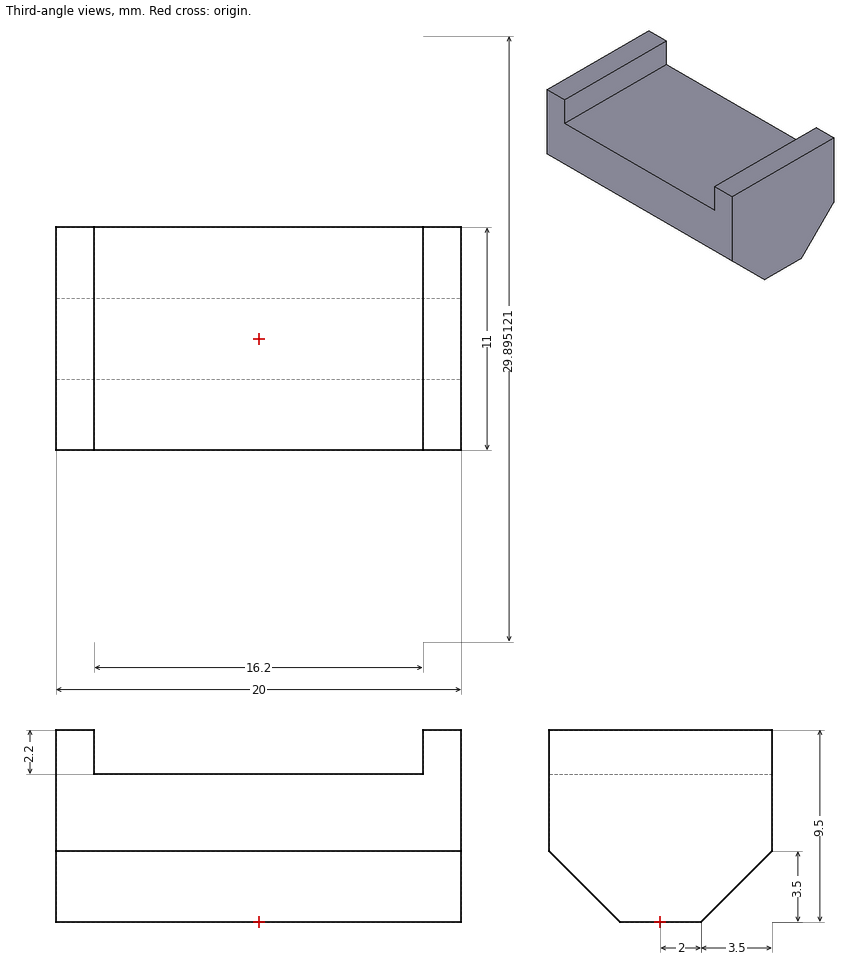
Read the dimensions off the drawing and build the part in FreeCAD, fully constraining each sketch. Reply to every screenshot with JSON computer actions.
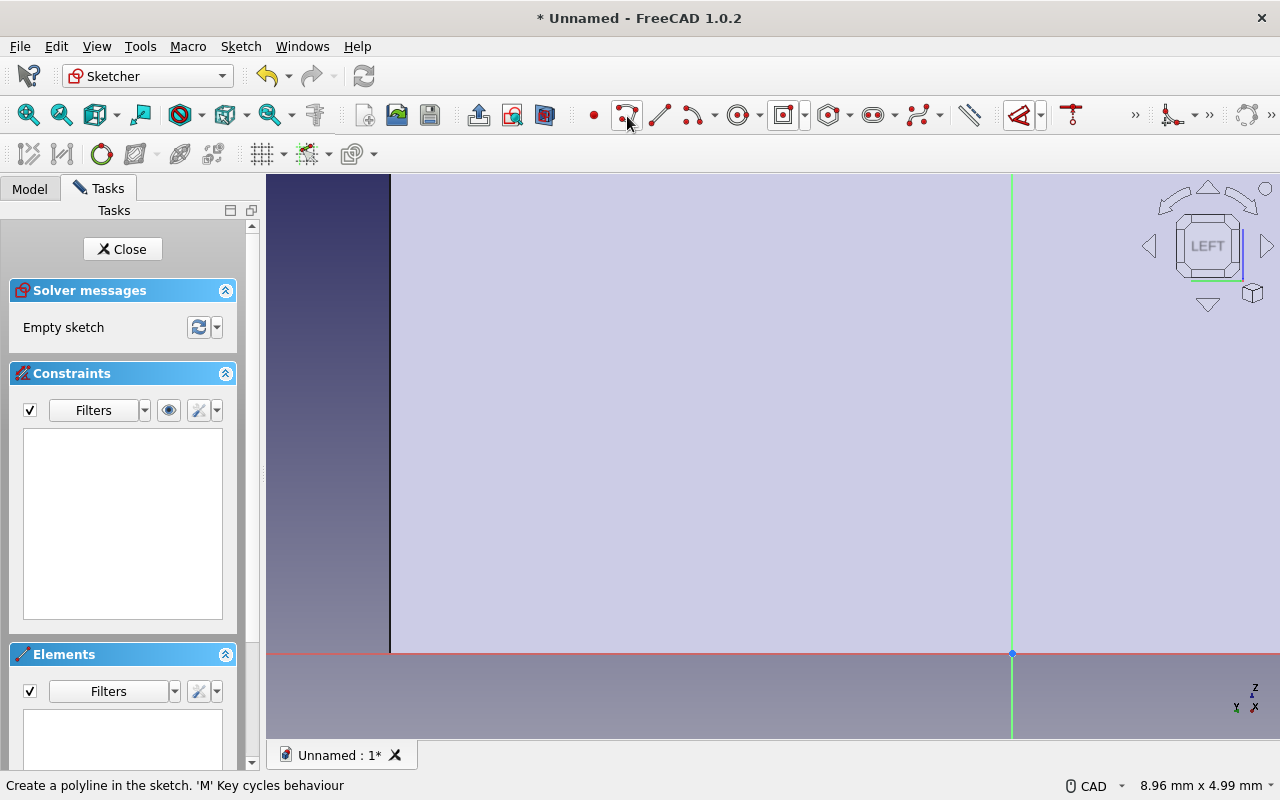
{"action": "left_click", "coordinate": [786, 654]}
{"action": "left_click", "coordinate": [390, 257]}
{"action": "left_click", "coordinate": [390, 645]}
{"action": "left_click", "coordinate": [786, 654]}
{"action": "key", "text": "Escape"}
{"action": "key", "text": "Escape"}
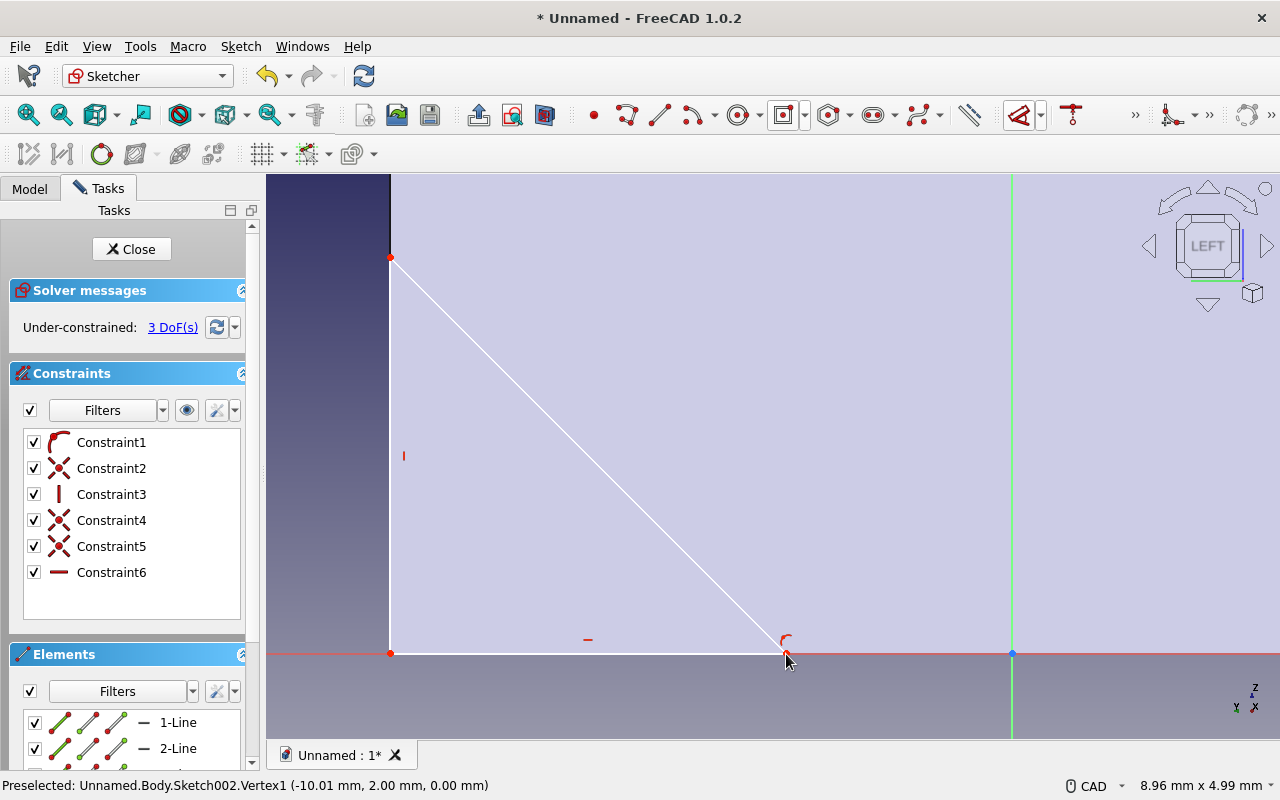
{"action": "left_click", "coordinate": [1018, 116]}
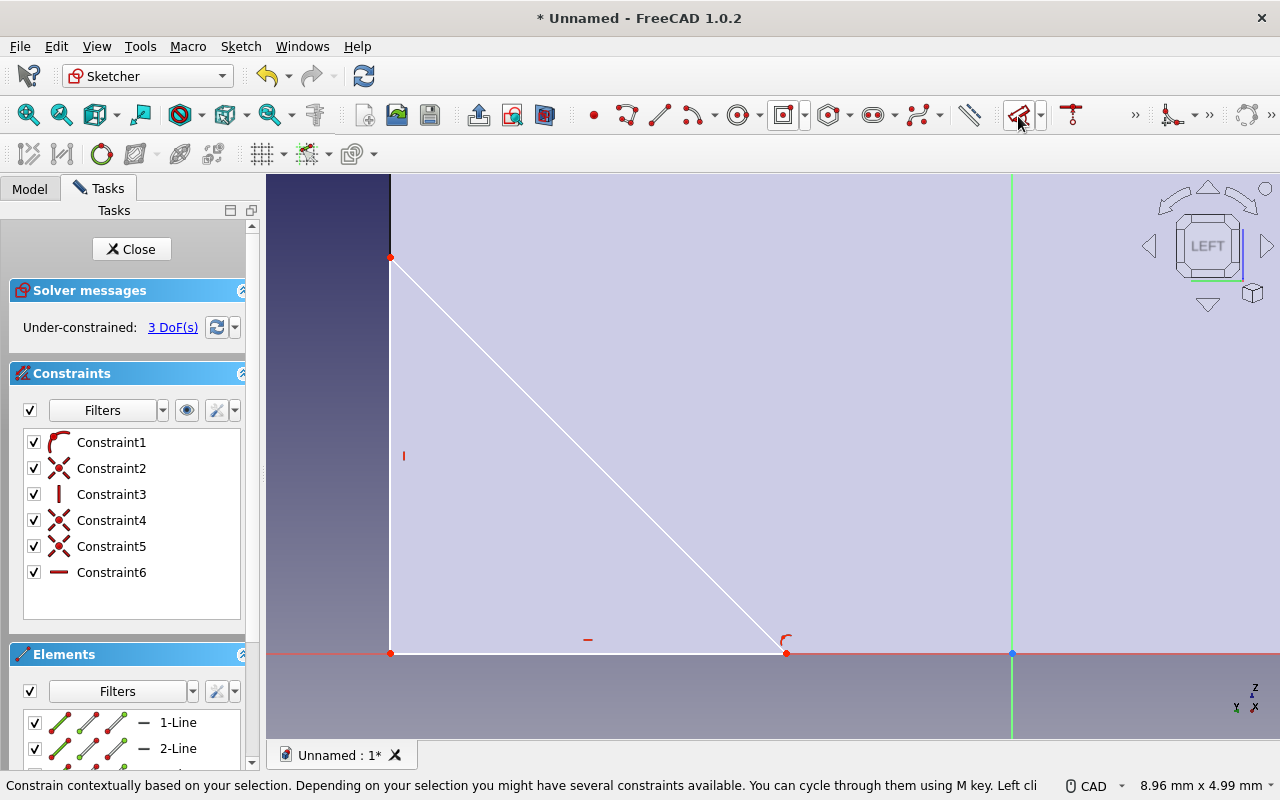
{"action": "left_click", "coordinate": [786, 654]}
{"action": "left_click", "coordinate": [899, 688]}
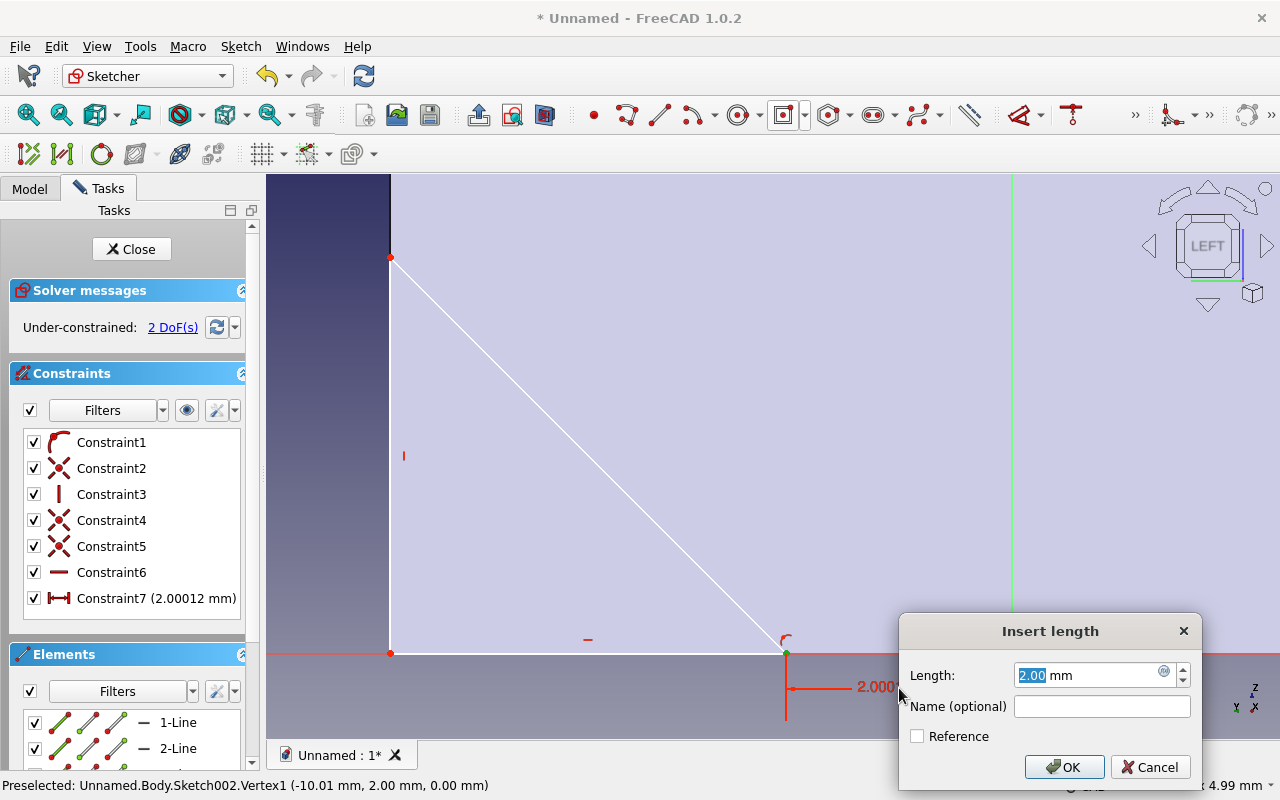
{"action": "type", "text": "2"}
{"action": "key", "text": "Return"}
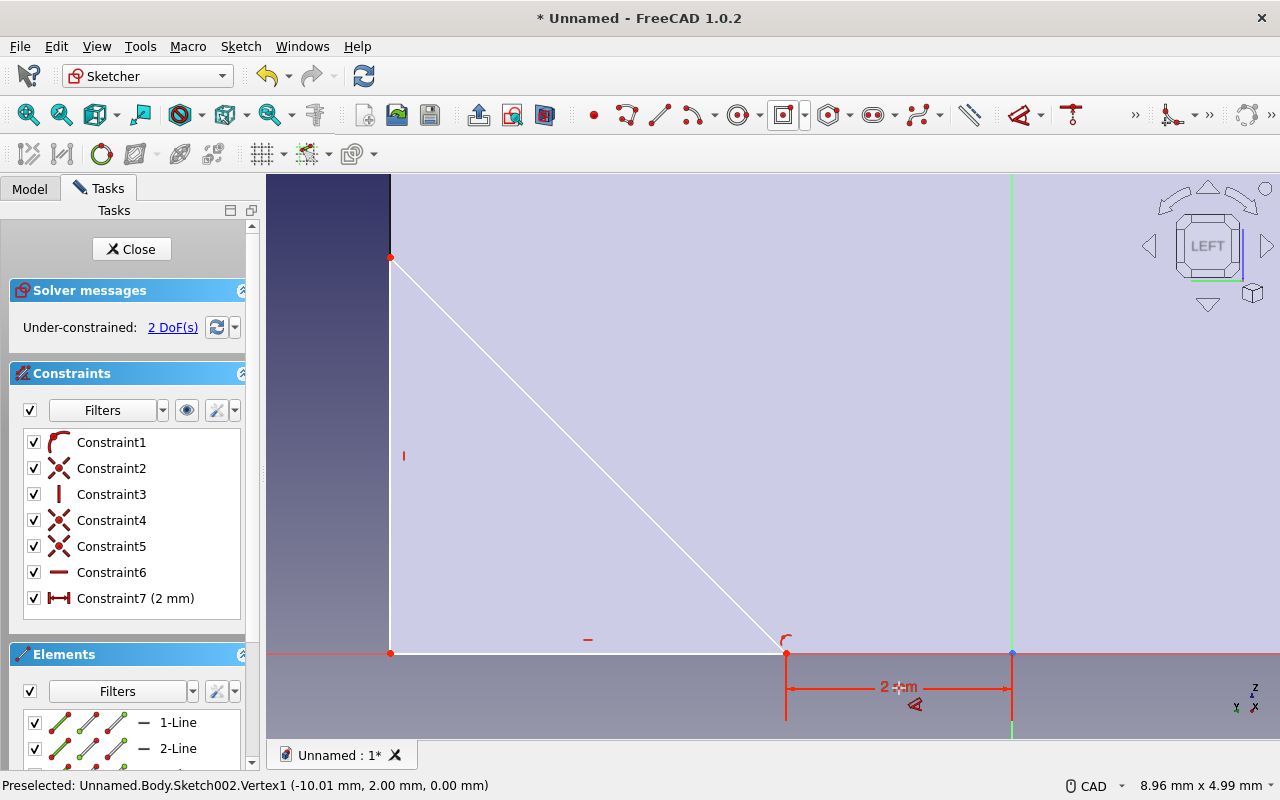
{"action": "left_click", "coordinate": [390, 377]}
{"action": "left_click", "coordinate": [356, 456]}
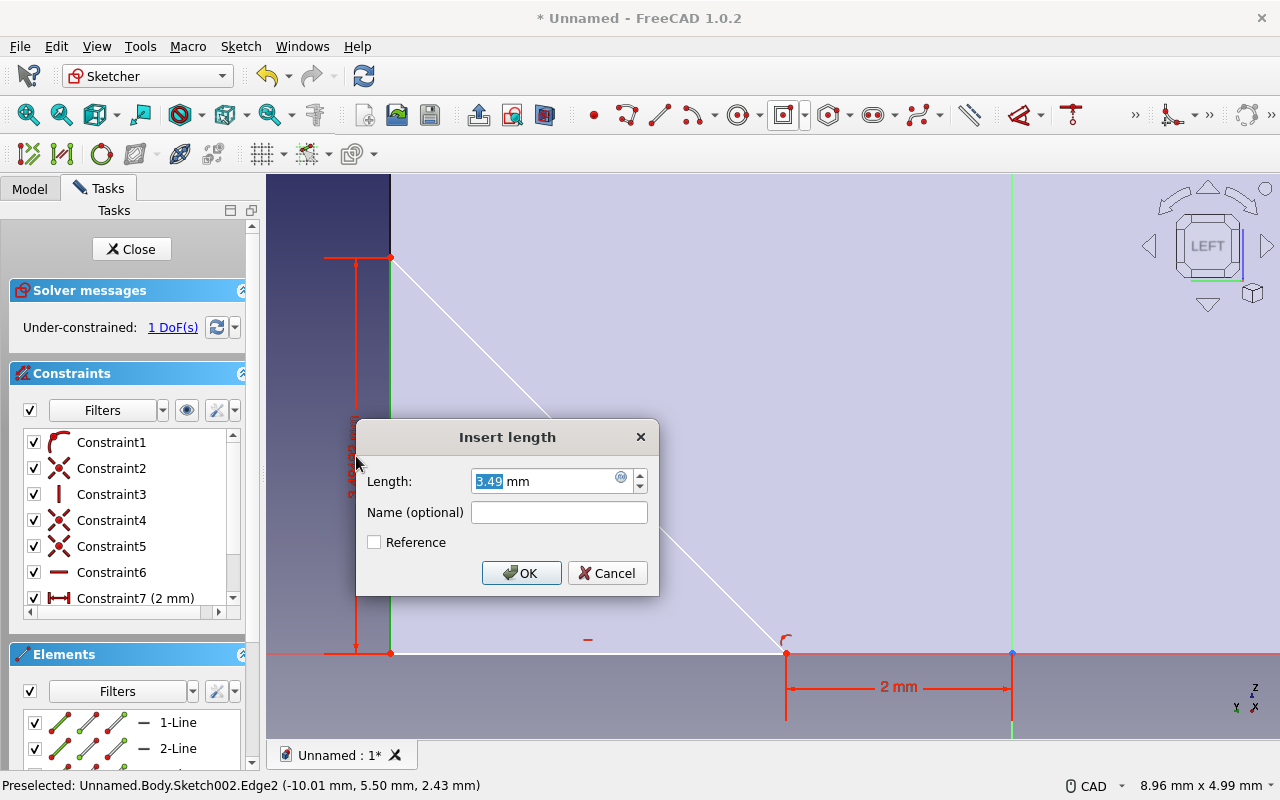
{"action": "type", "text": "3.5"}
{"action": "key", "text": "Return"}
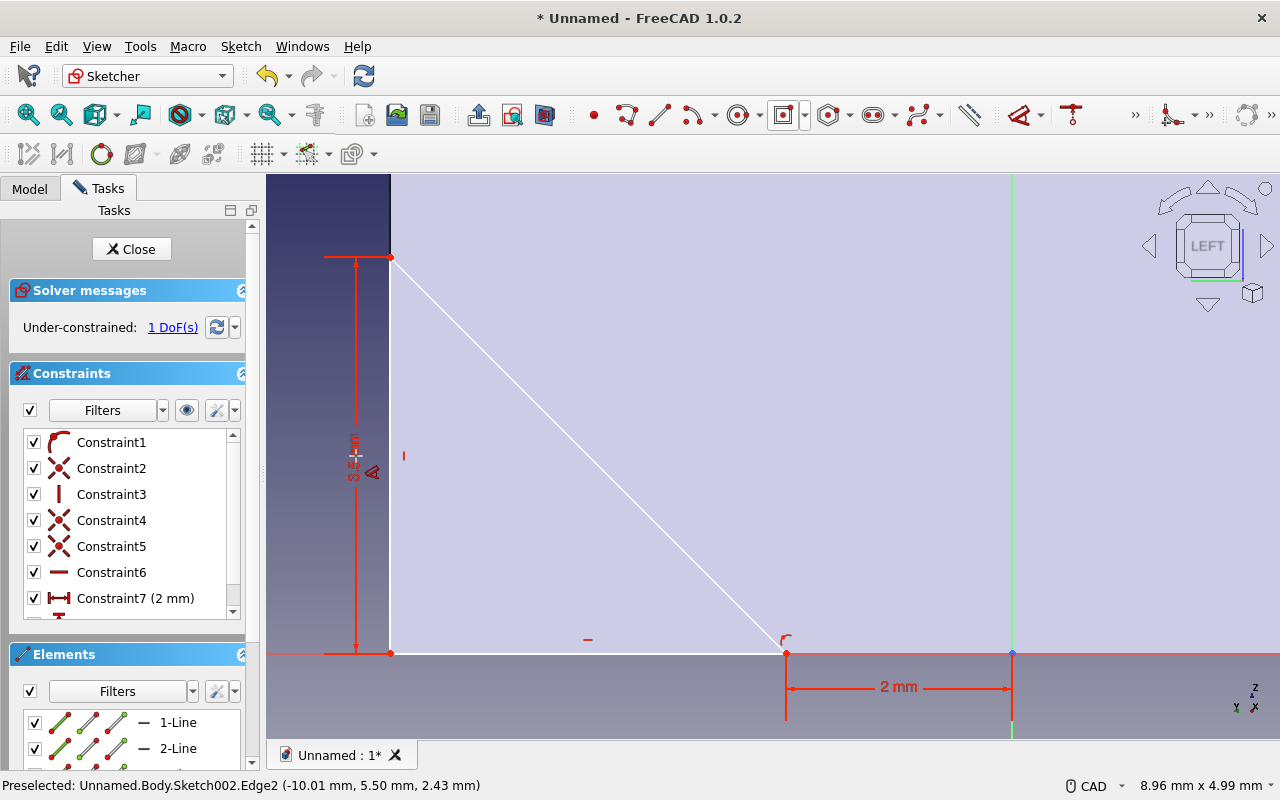
{"action": "left_click", "coordinate": [509, 654]}
{"action": "left_click", "coordinate": [588, 688]}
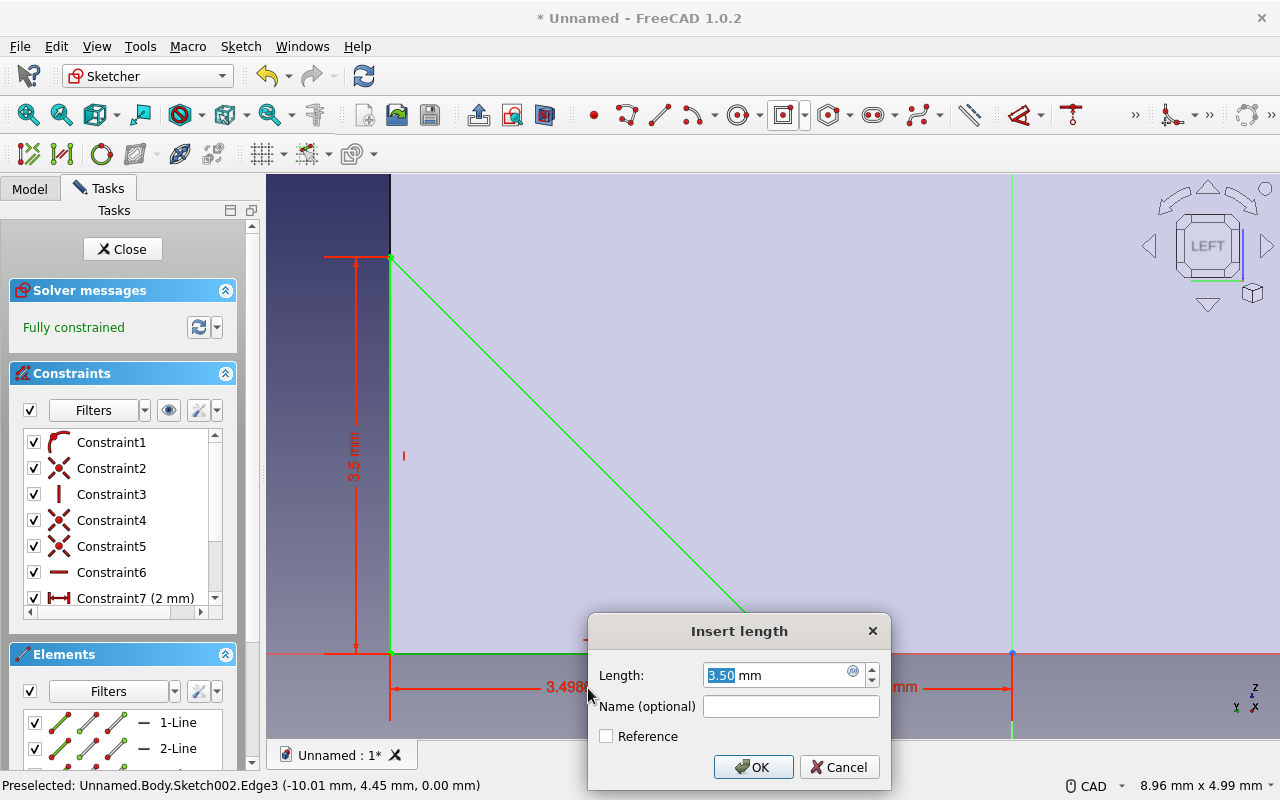
{"action": "type", "text": "3.5"}
{"action": "key", "text": "Return"}
{"action": "key", "text": "Escape"}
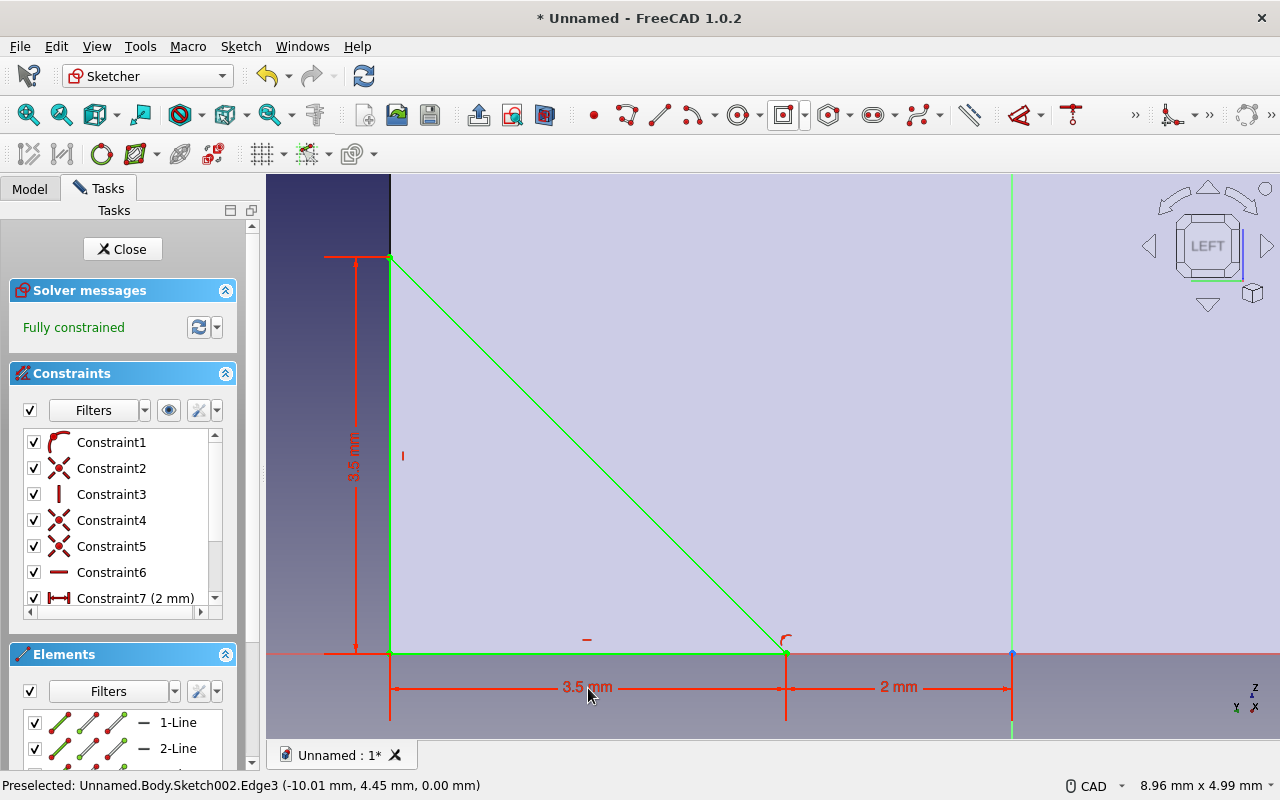
{"action": "left_click", "coordinate": [123, 249]}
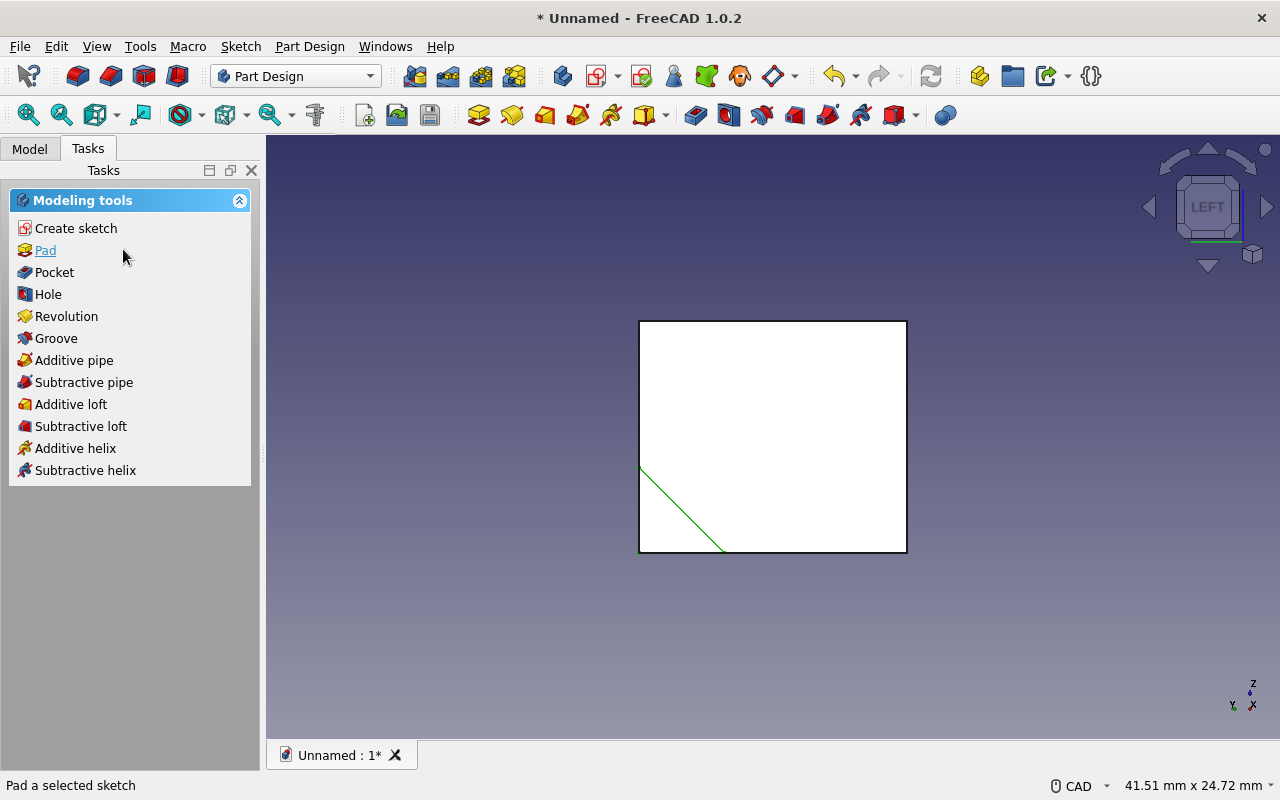
{"action": "left_click", "coordinate": [696, 116]}